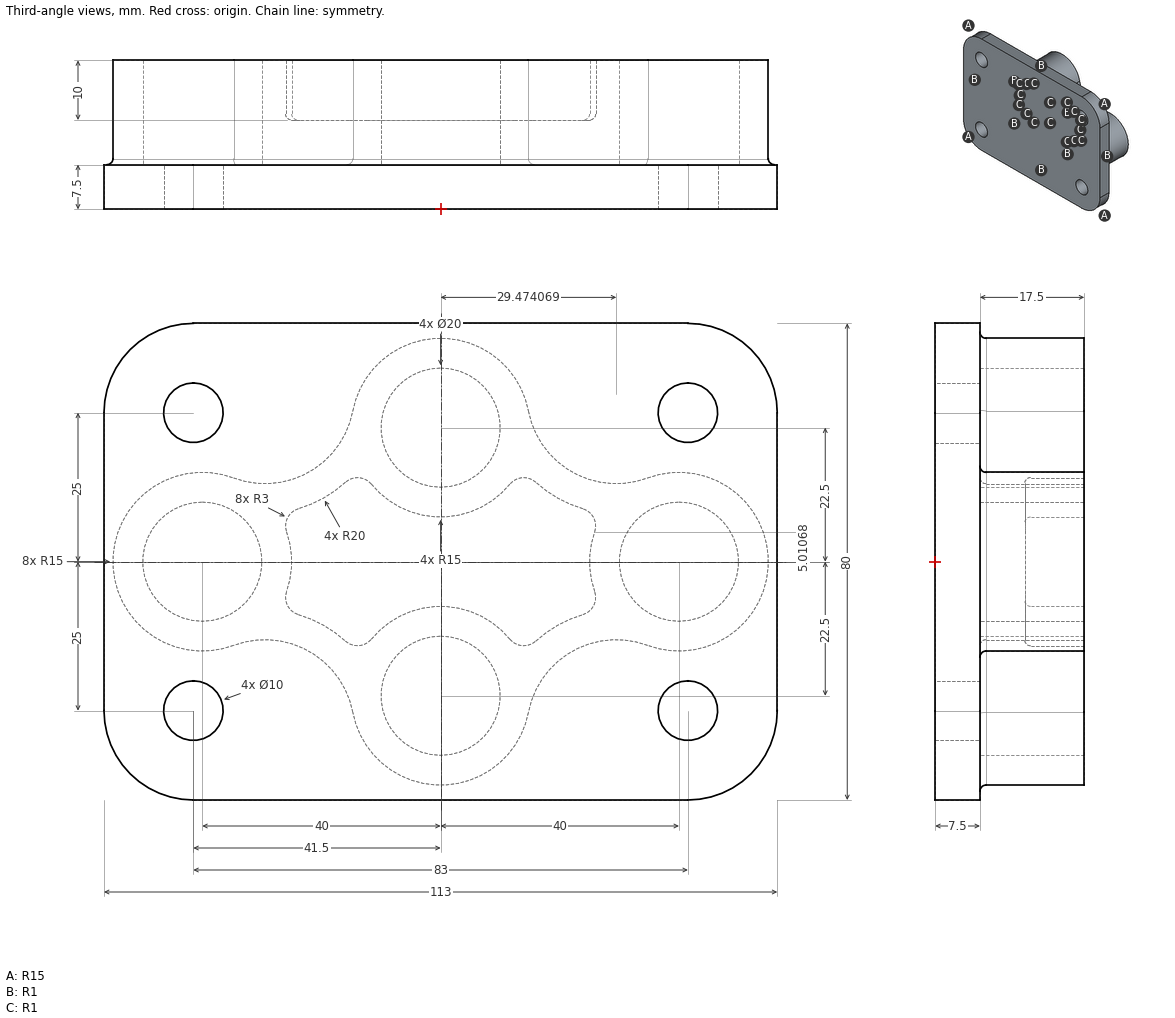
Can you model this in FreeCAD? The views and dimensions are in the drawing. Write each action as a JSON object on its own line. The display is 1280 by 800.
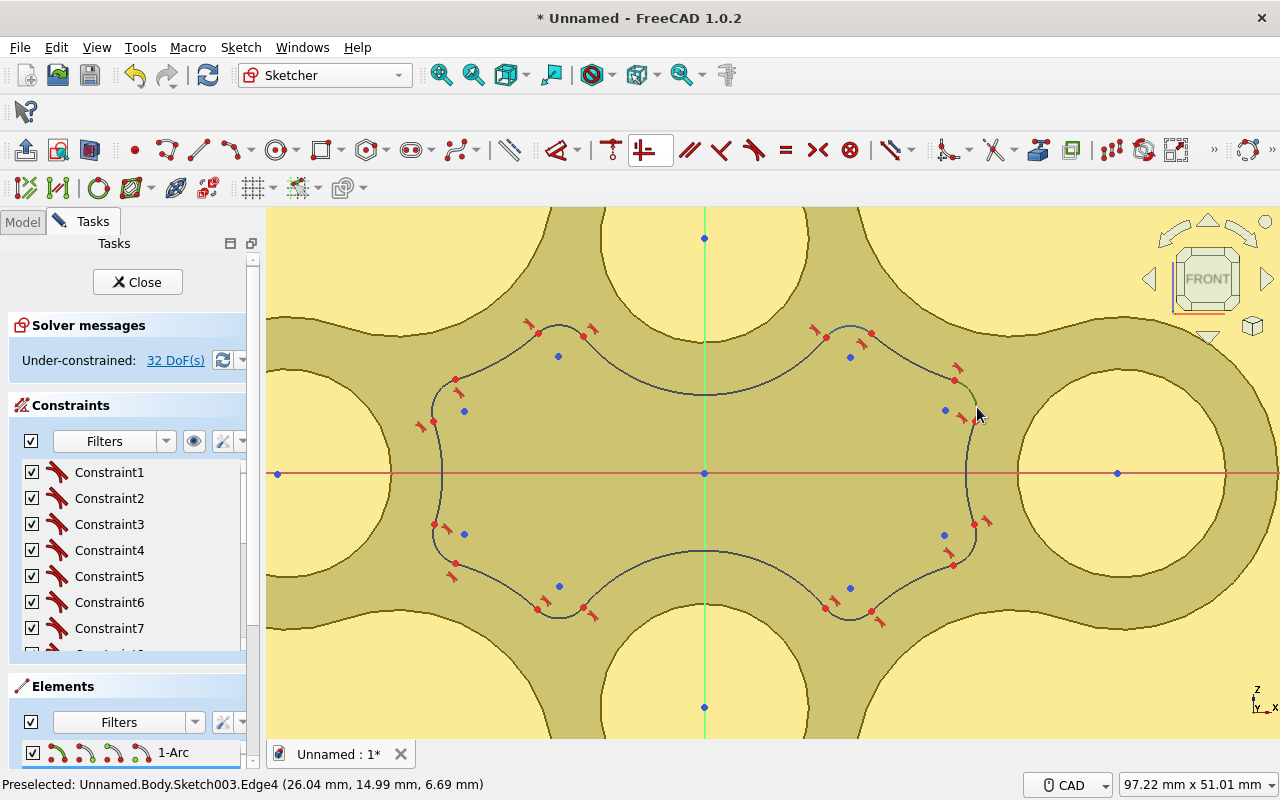
{"action": "left_click", "coordinate": [967, 558]}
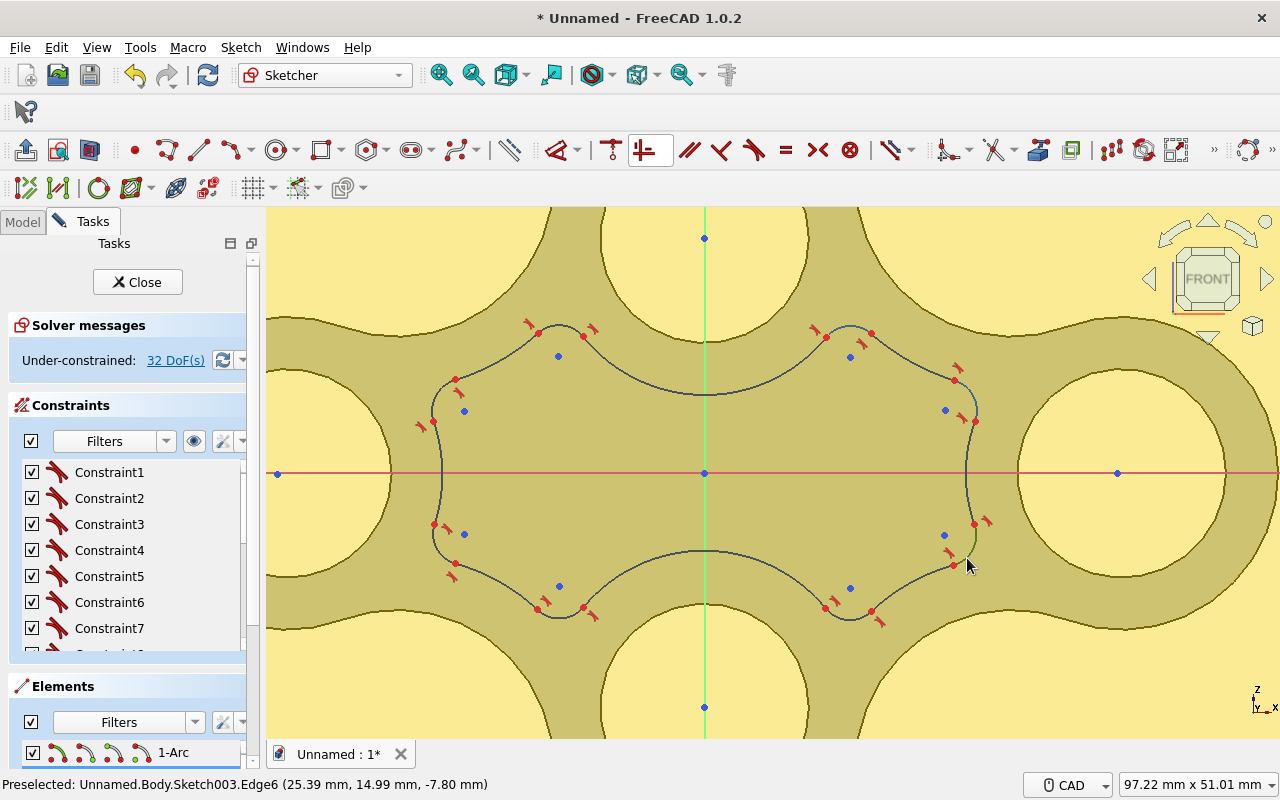
{"action": "left_click", "coordinate": [838, 618]}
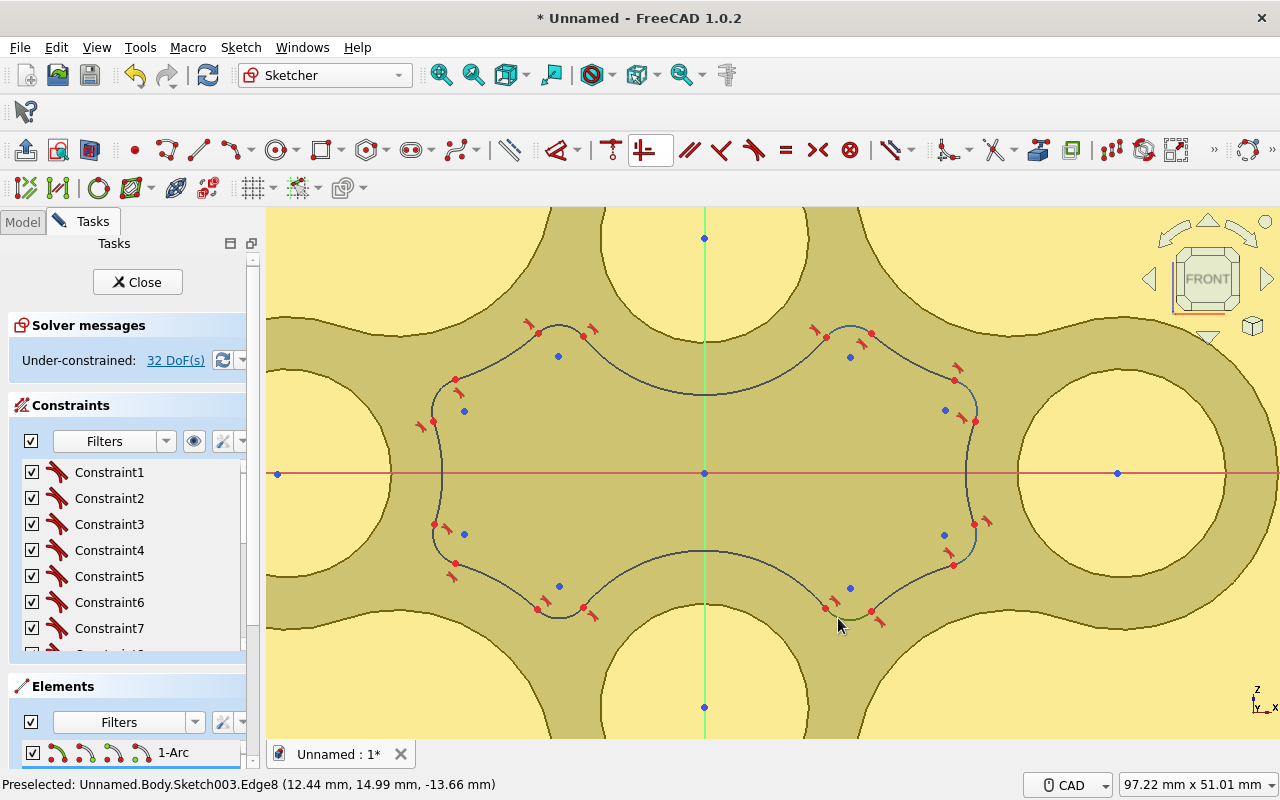
{"action": "left_click", "coordinate": [551, 617]}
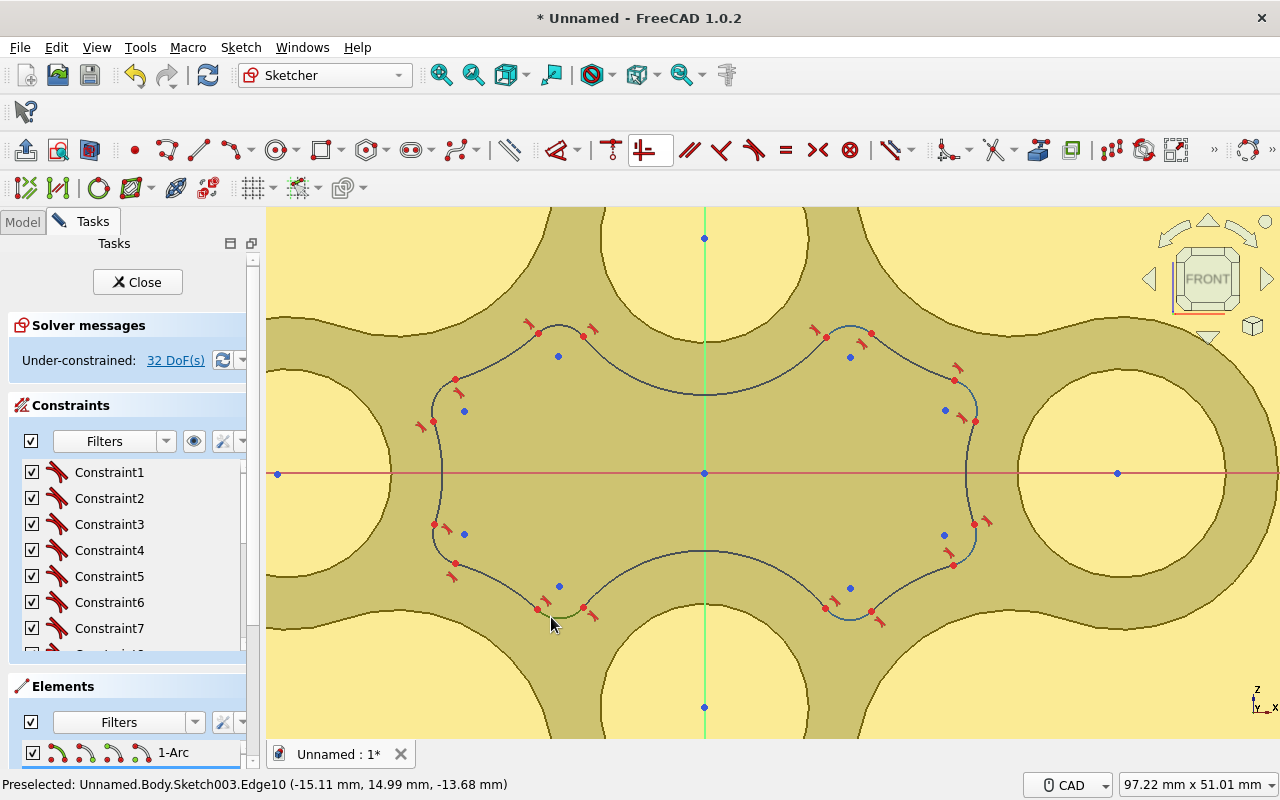
{"action": "left_click", "coordinate": [434, 539]}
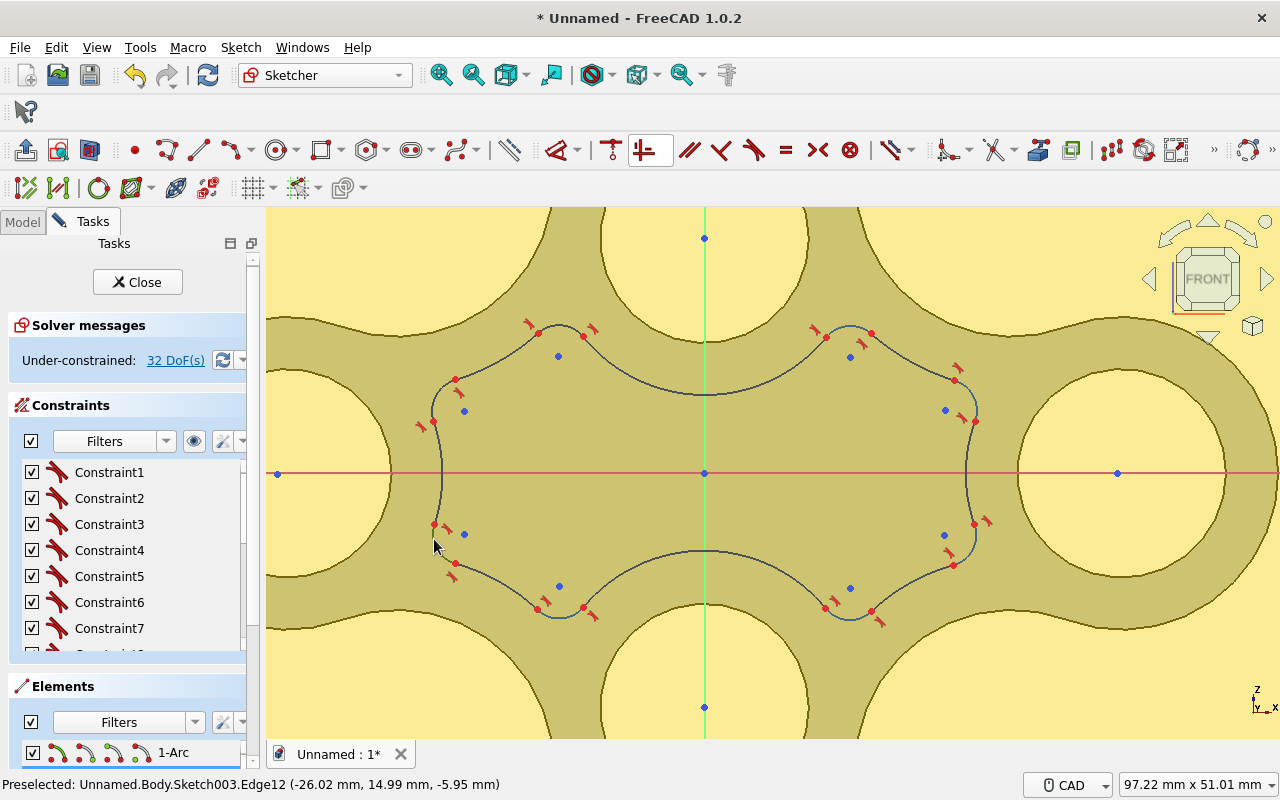
{"action": "left_click", "coordinate": [442, 388]}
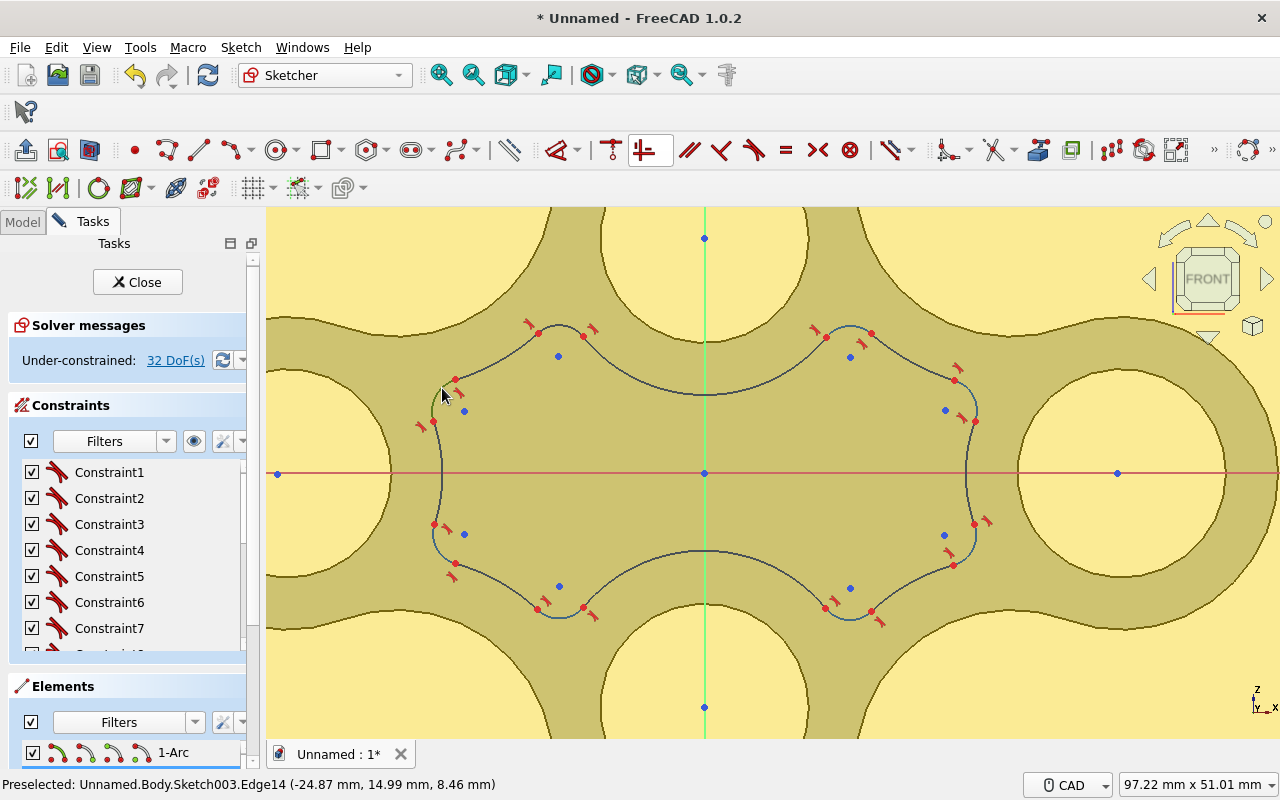
{"action": "left_click", "coordinate": [571, 328]}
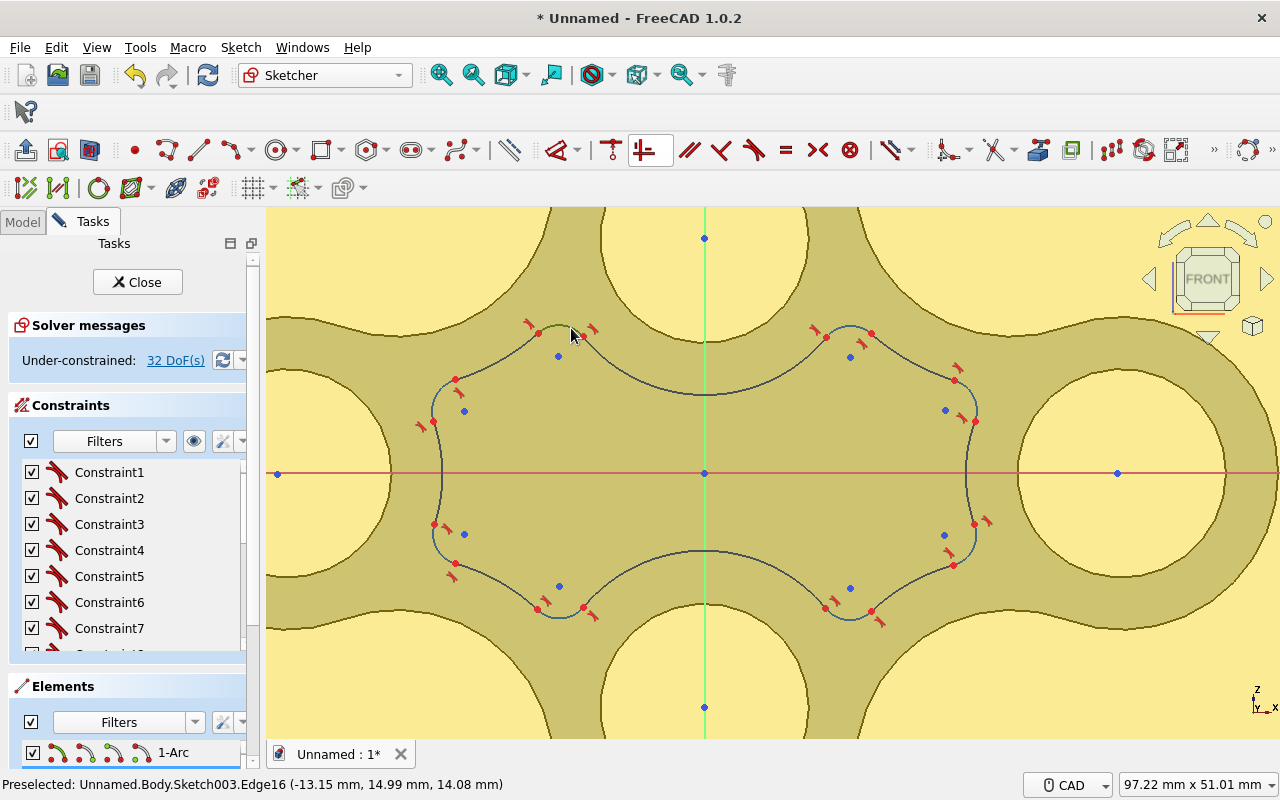
{"action": "key", "text": "e"}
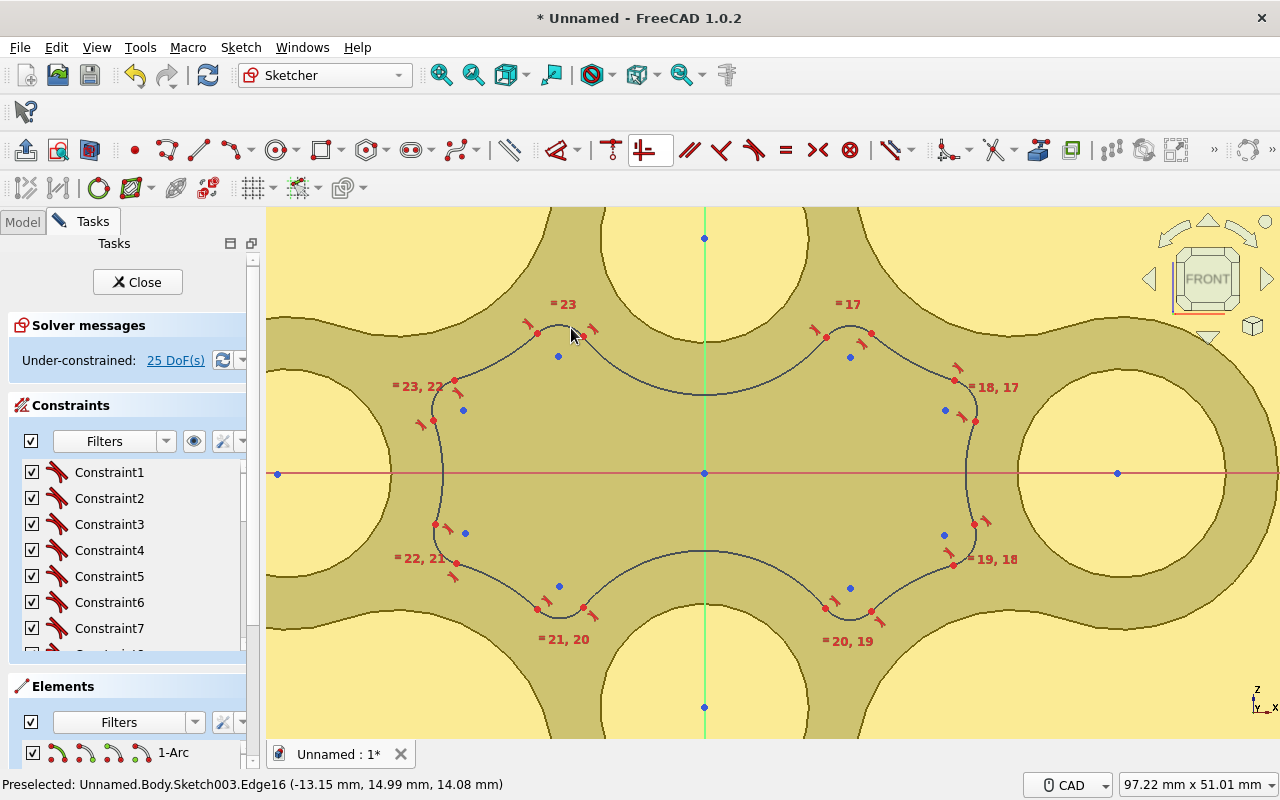
{"action": "left_click", "coordinate": [650, 385]}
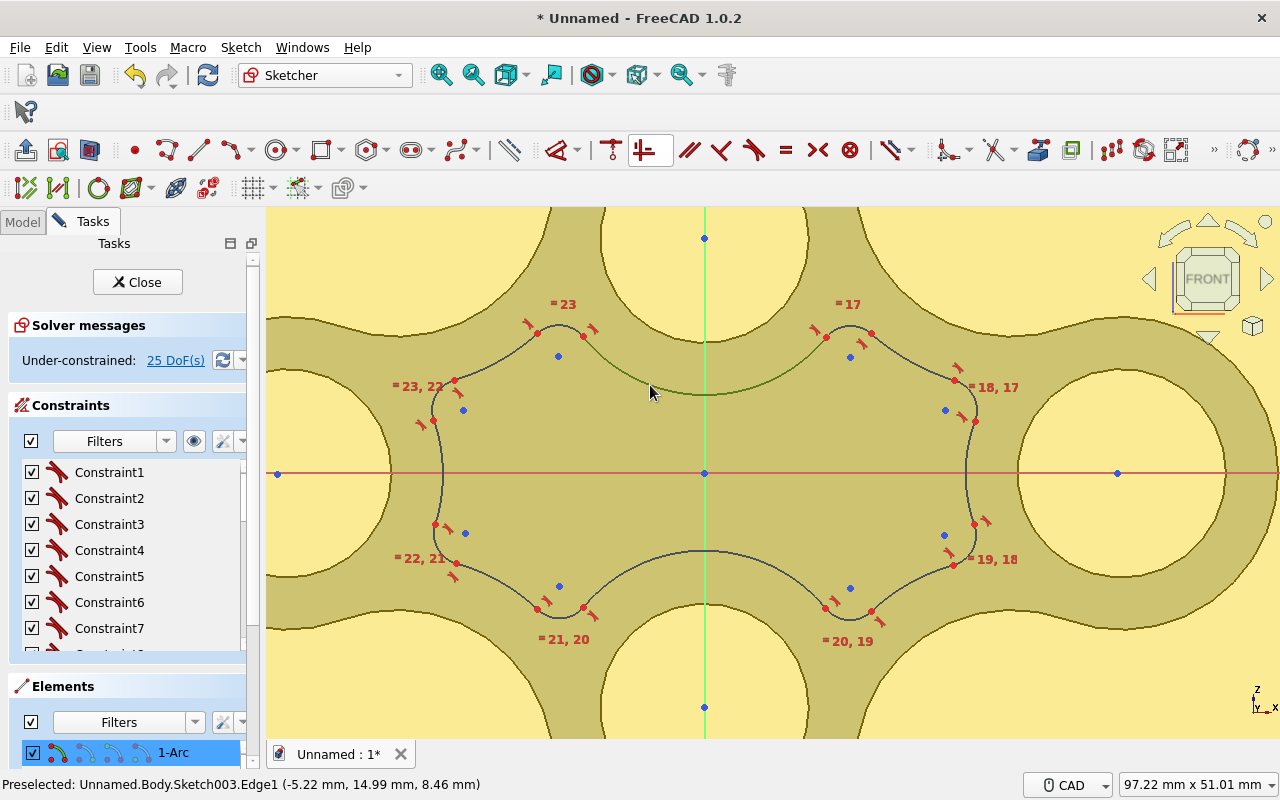
{"action": "left_click", "coordinate": [967, 452]}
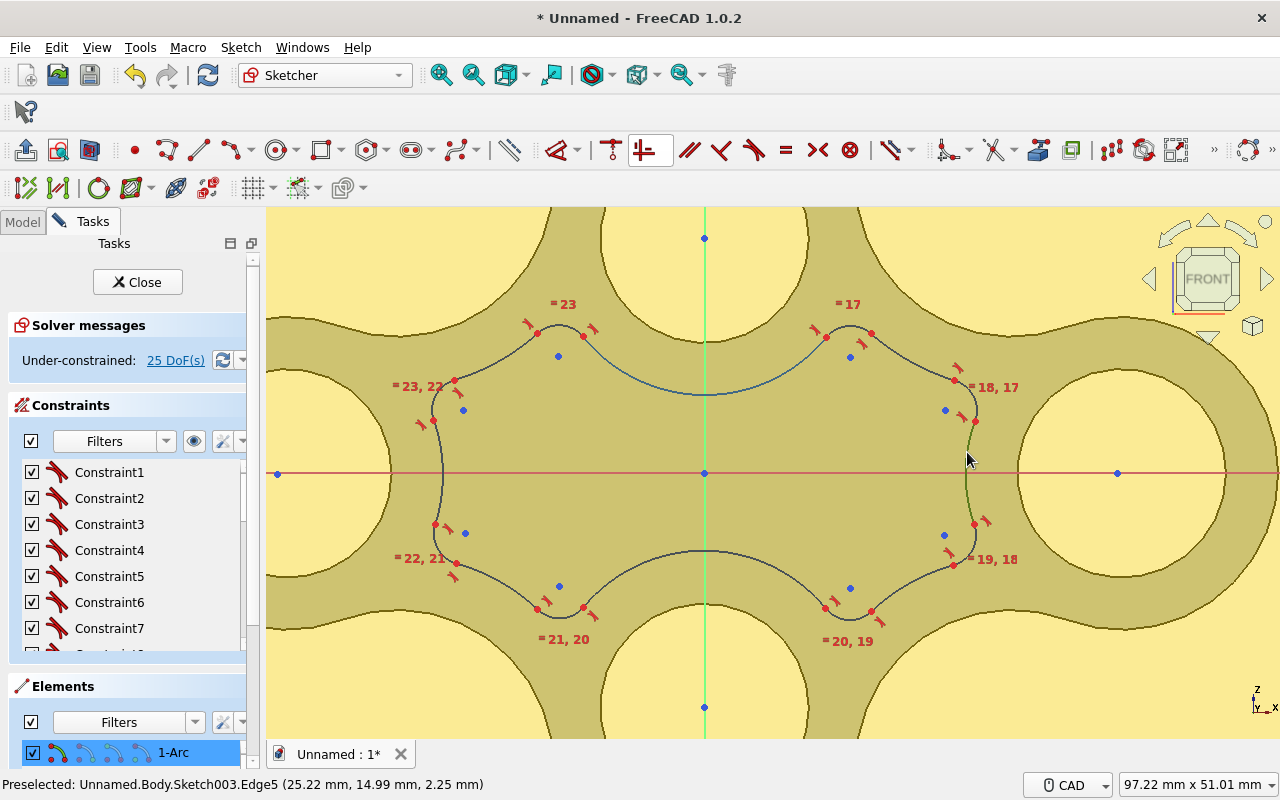
{"action": "left_click", "coordinate": [759, 561]}